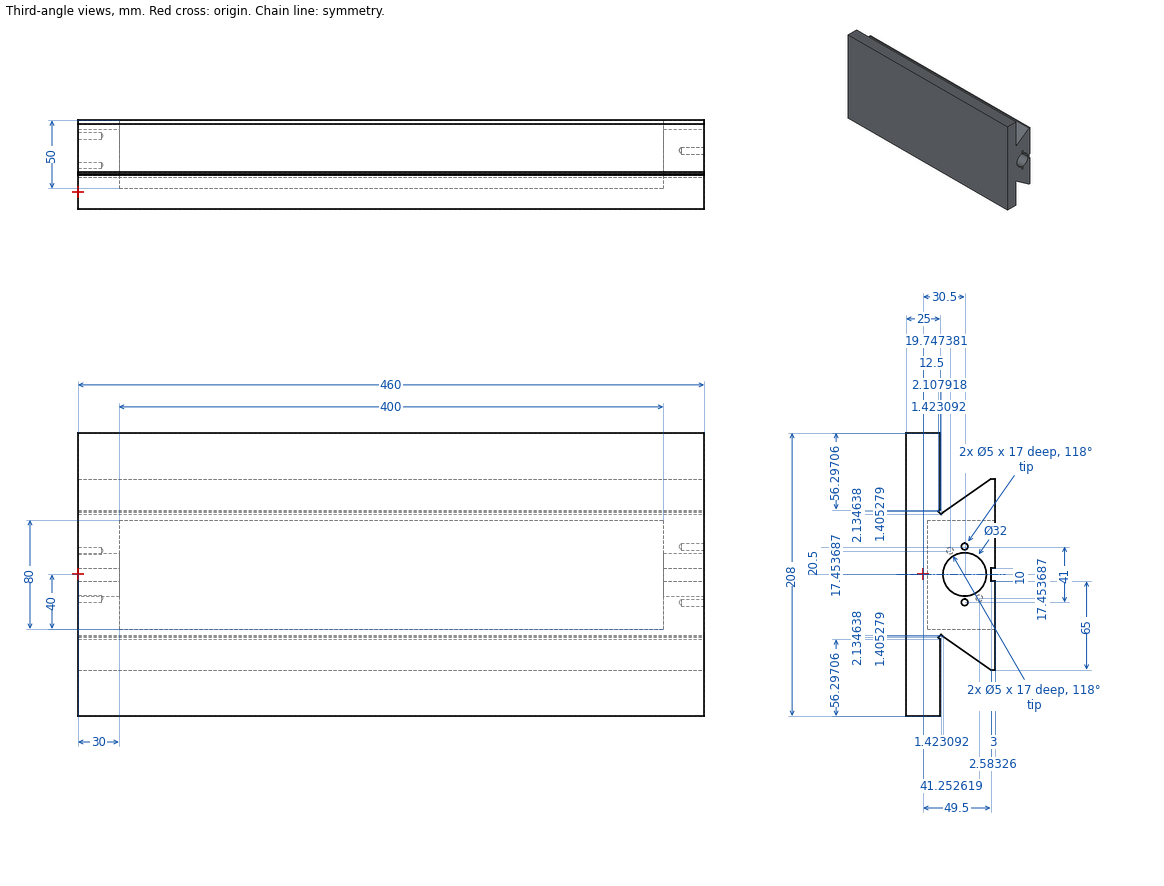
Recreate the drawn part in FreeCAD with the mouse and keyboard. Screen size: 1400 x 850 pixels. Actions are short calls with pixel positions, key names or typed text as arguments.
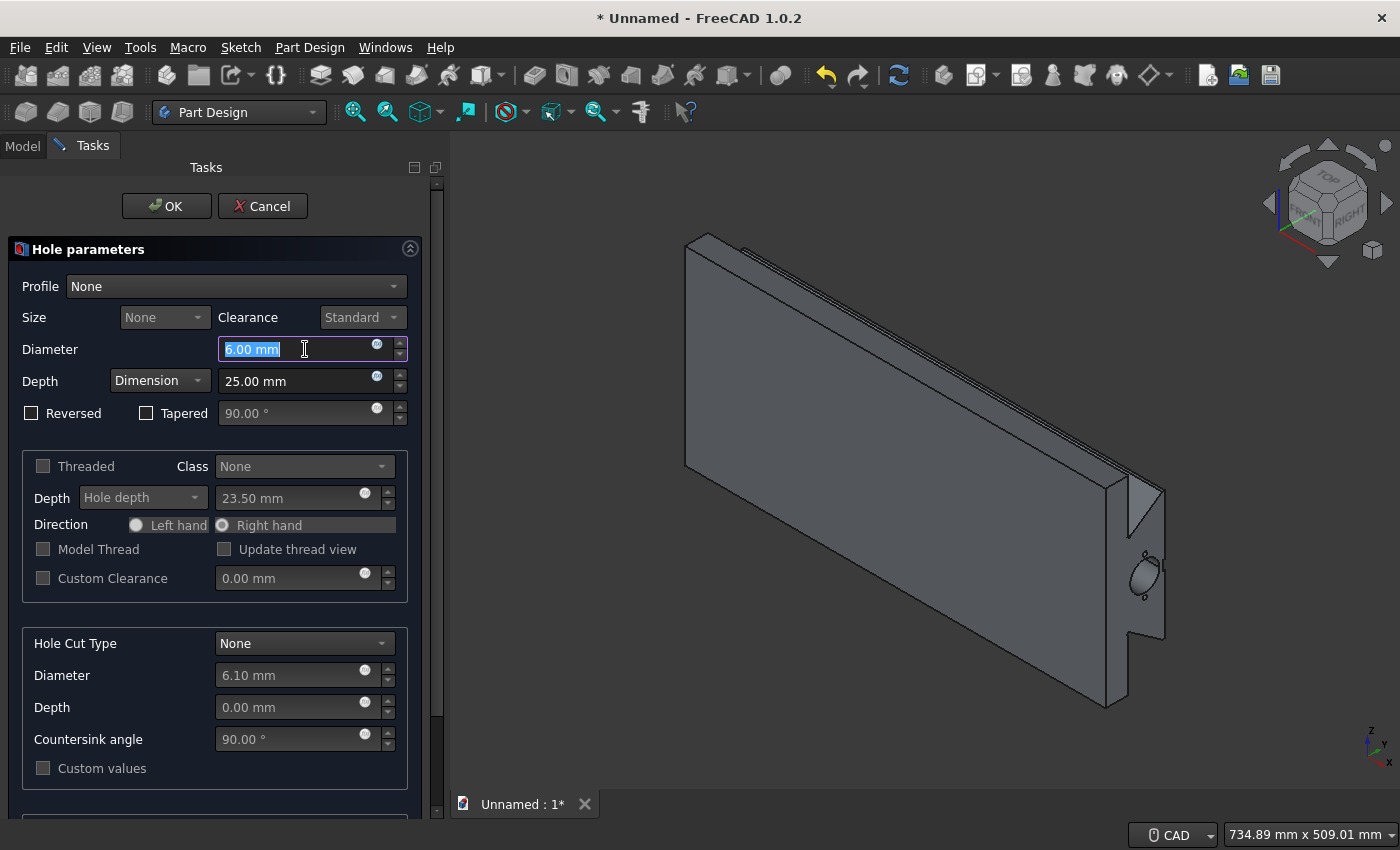
text(5)
key(Tab)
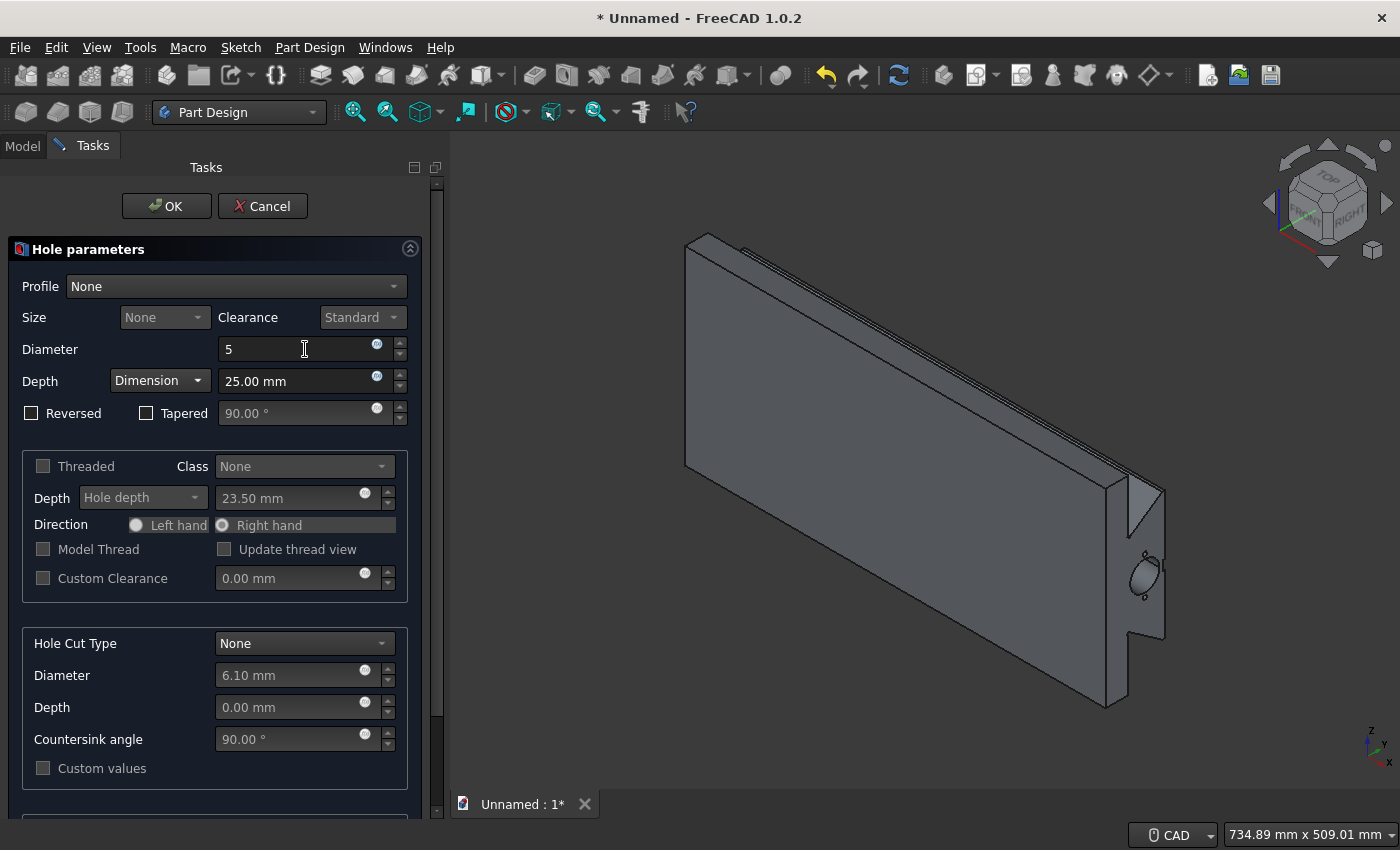
triple_click(305, 381)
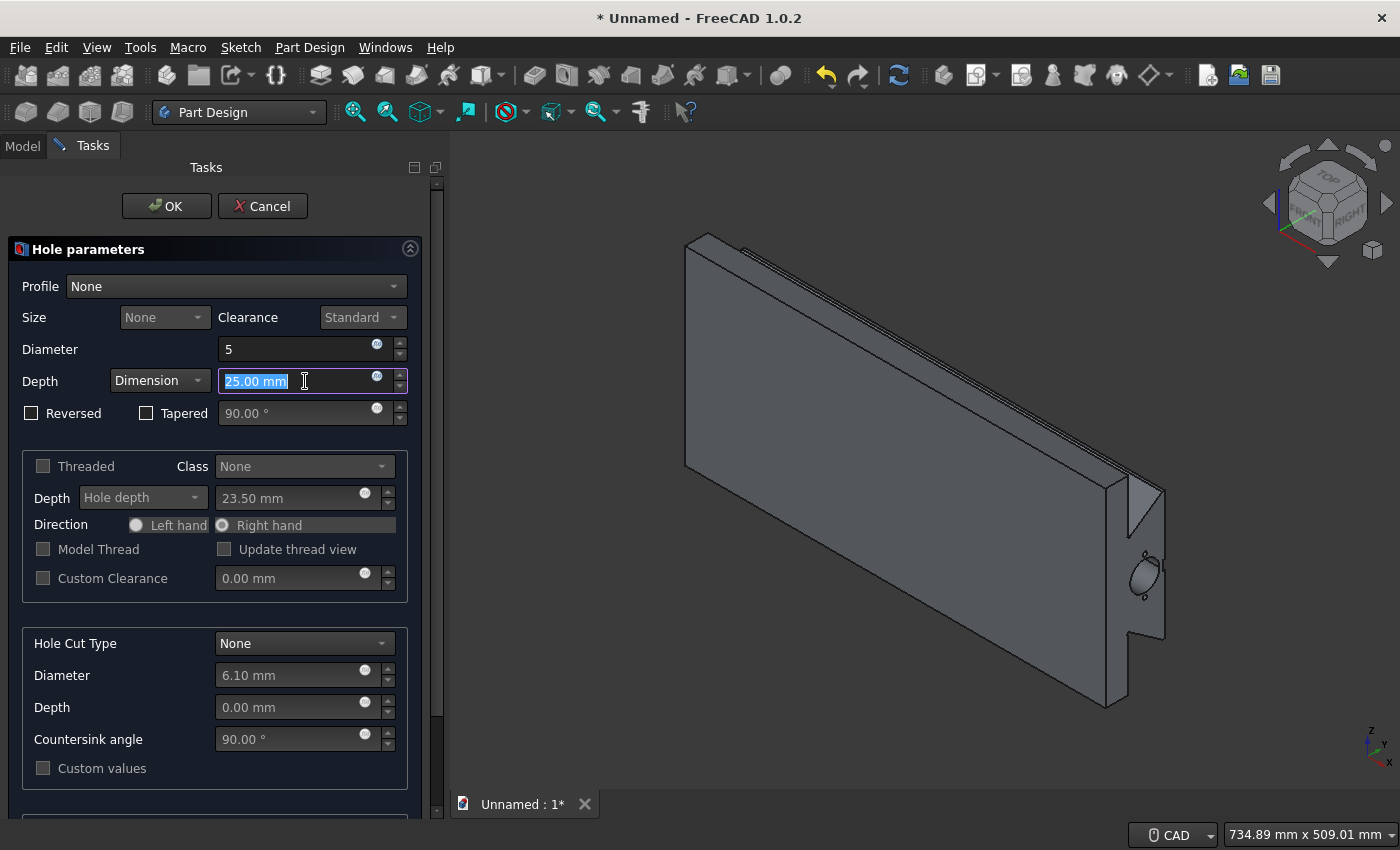
text(17)
key(Tab)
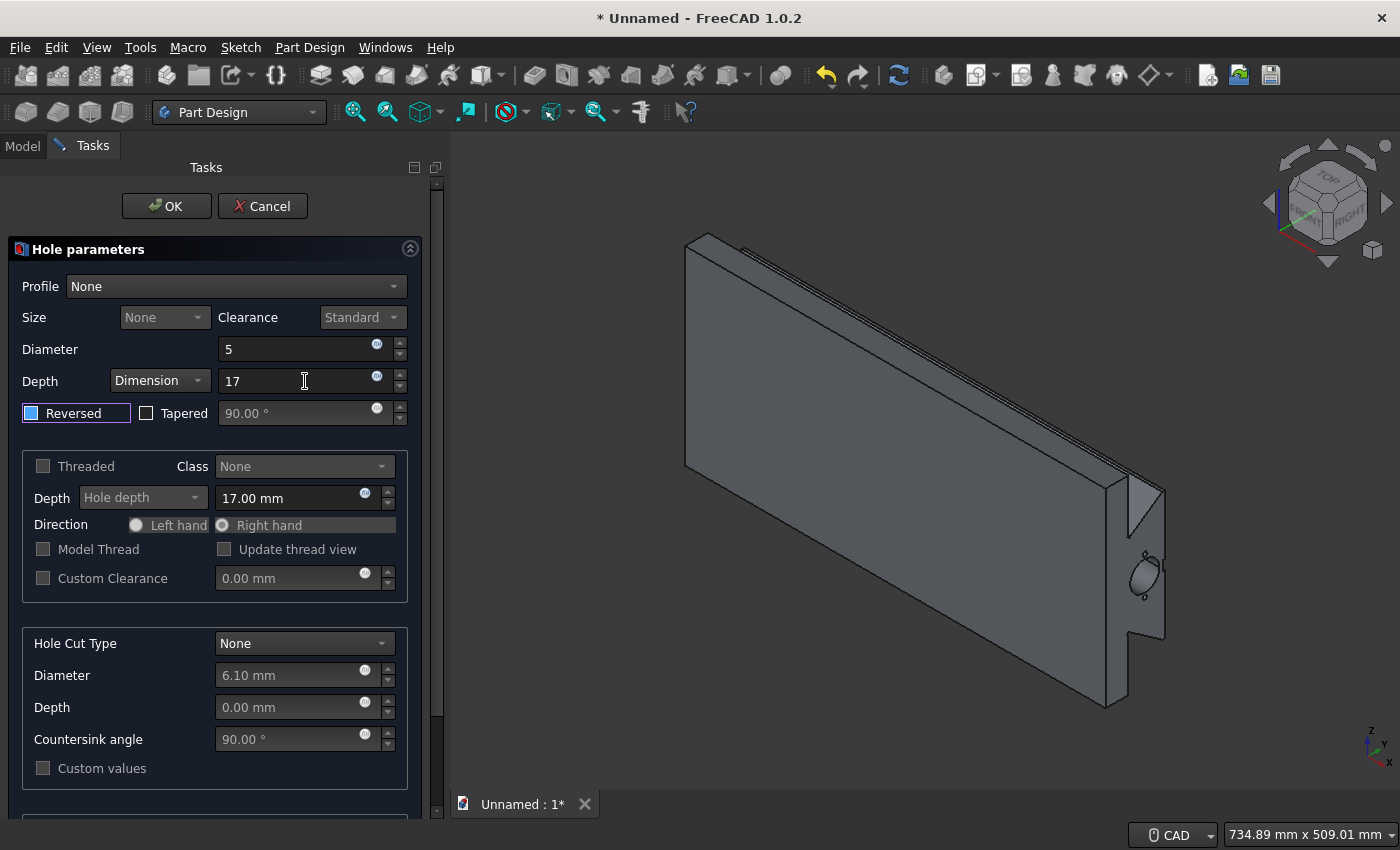
click(30, 413)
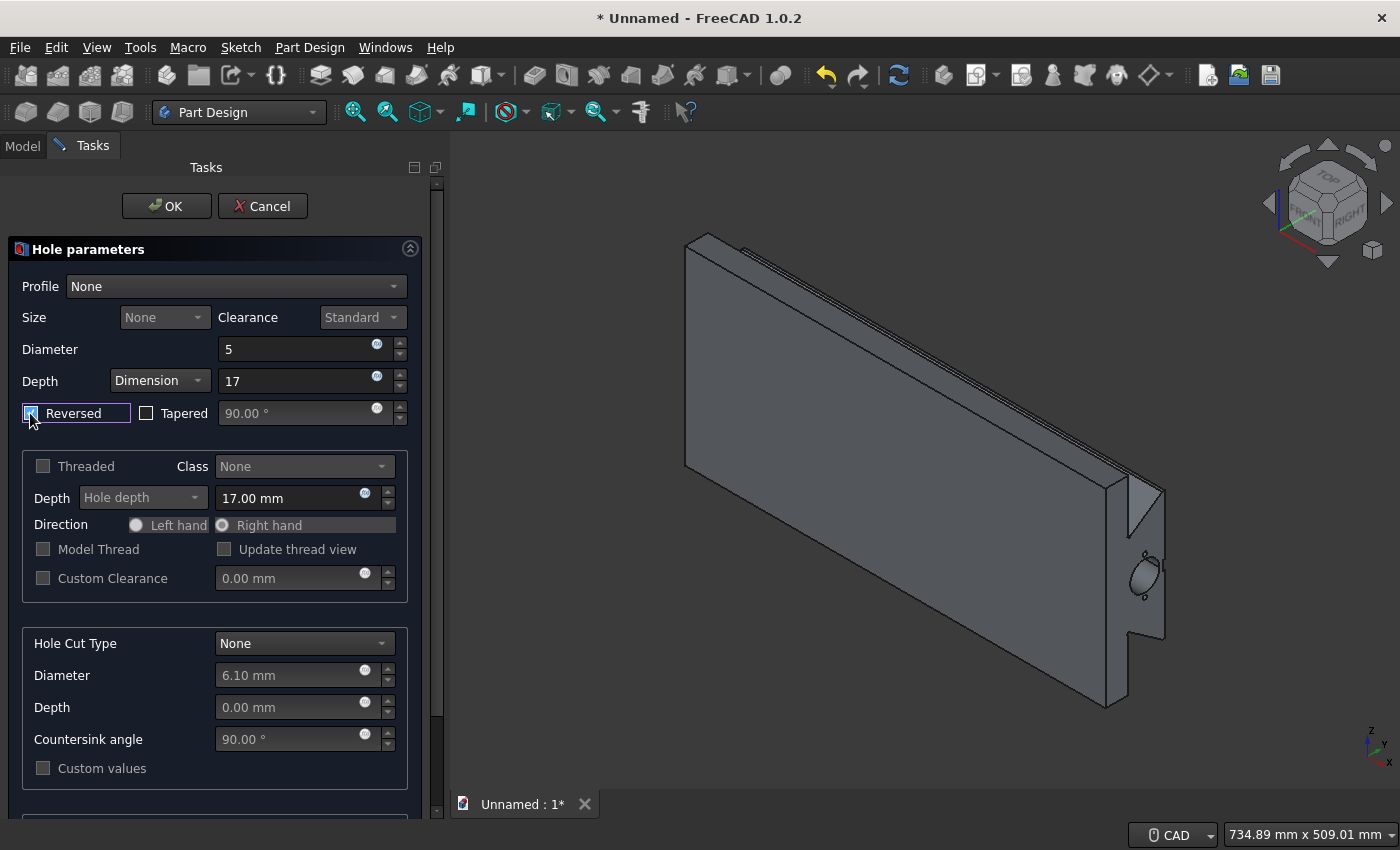
click(167, 206)